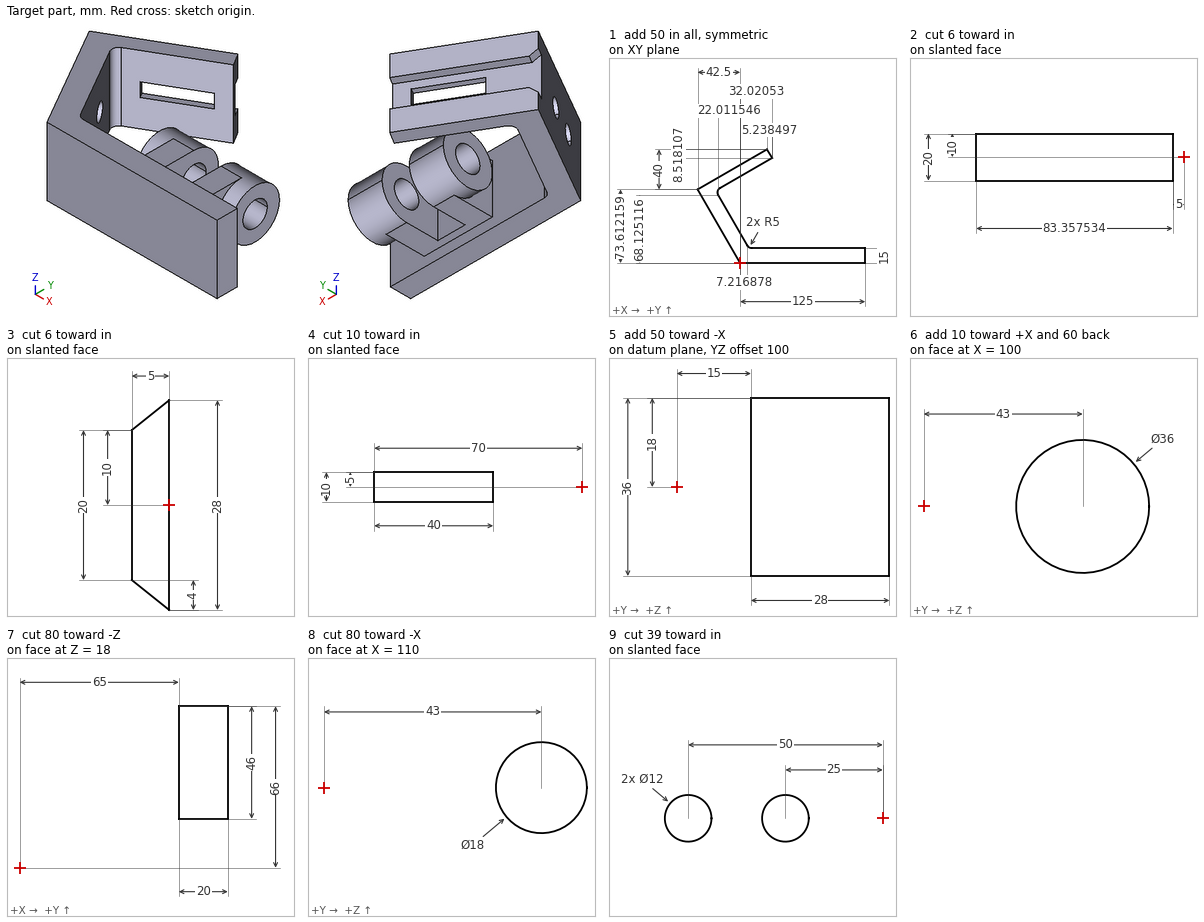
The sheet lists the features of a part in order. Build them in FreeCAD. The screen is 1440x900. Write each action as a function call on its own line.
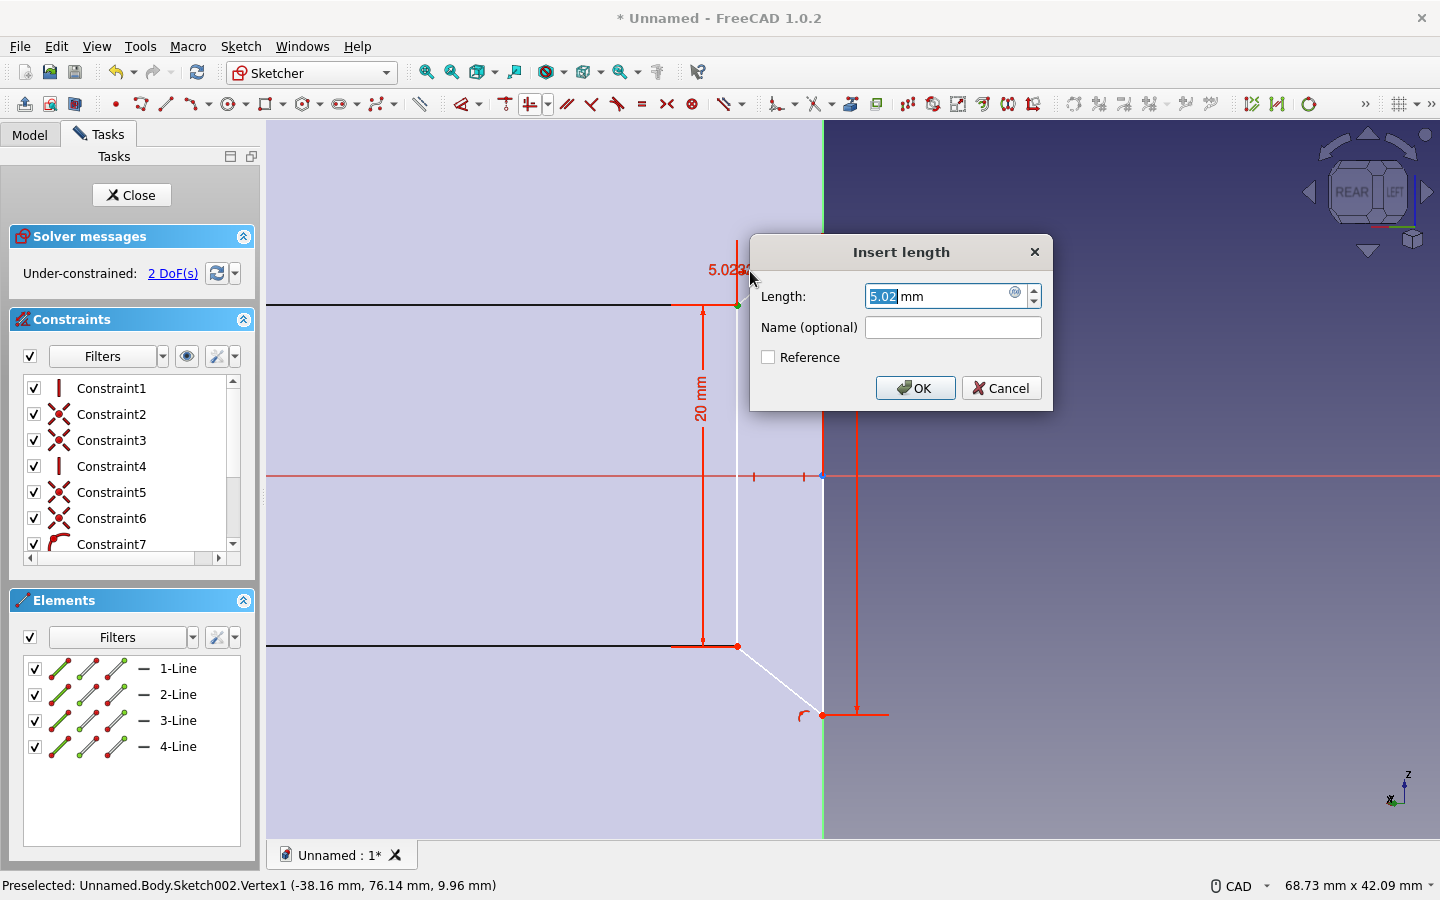
text(5)
key(Return)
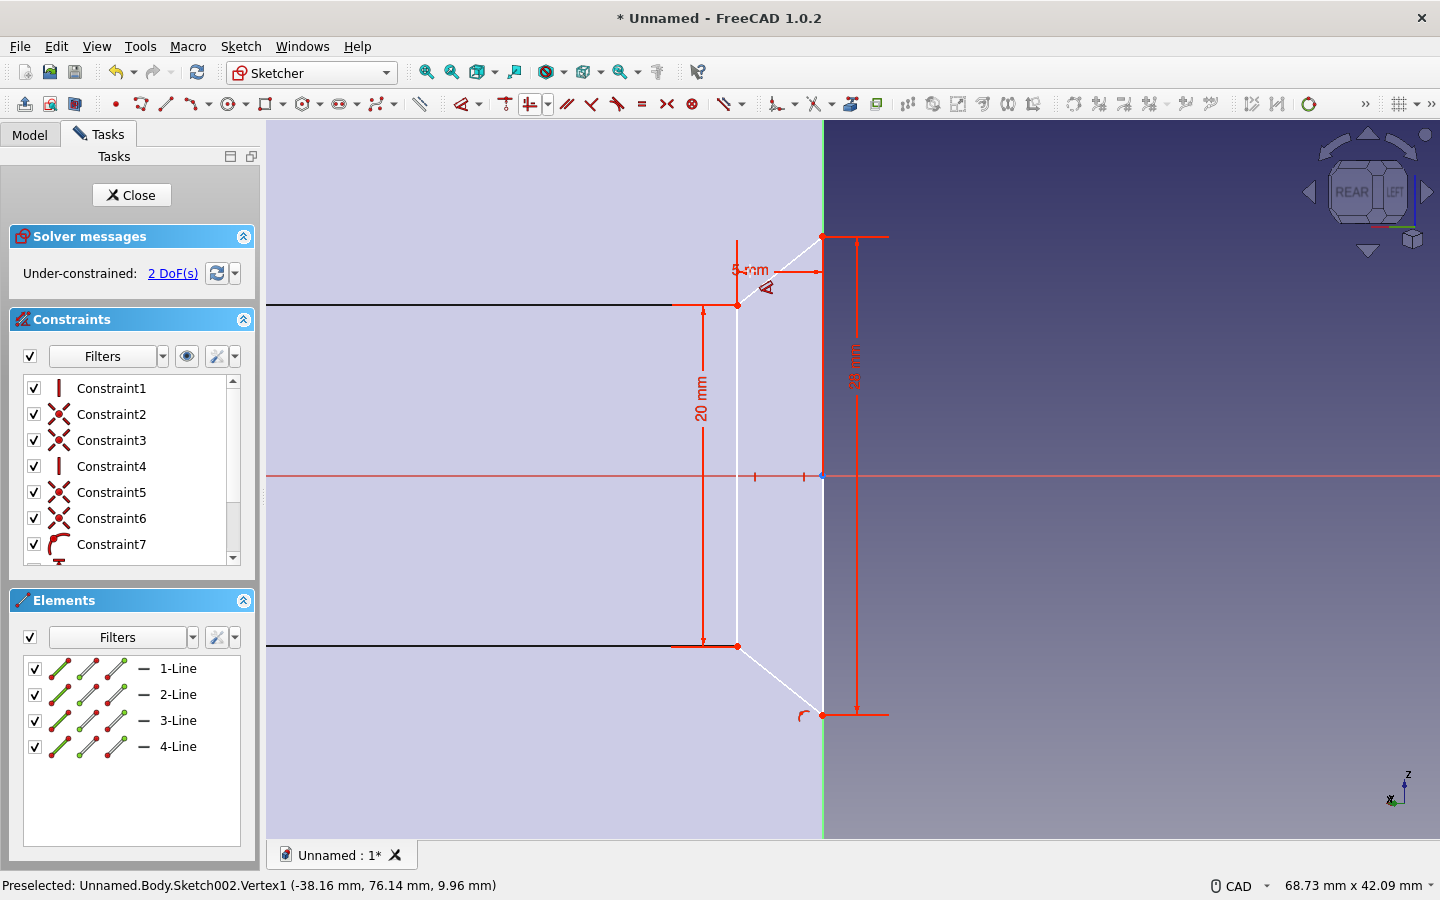
click(763, 667)
click(703, 681)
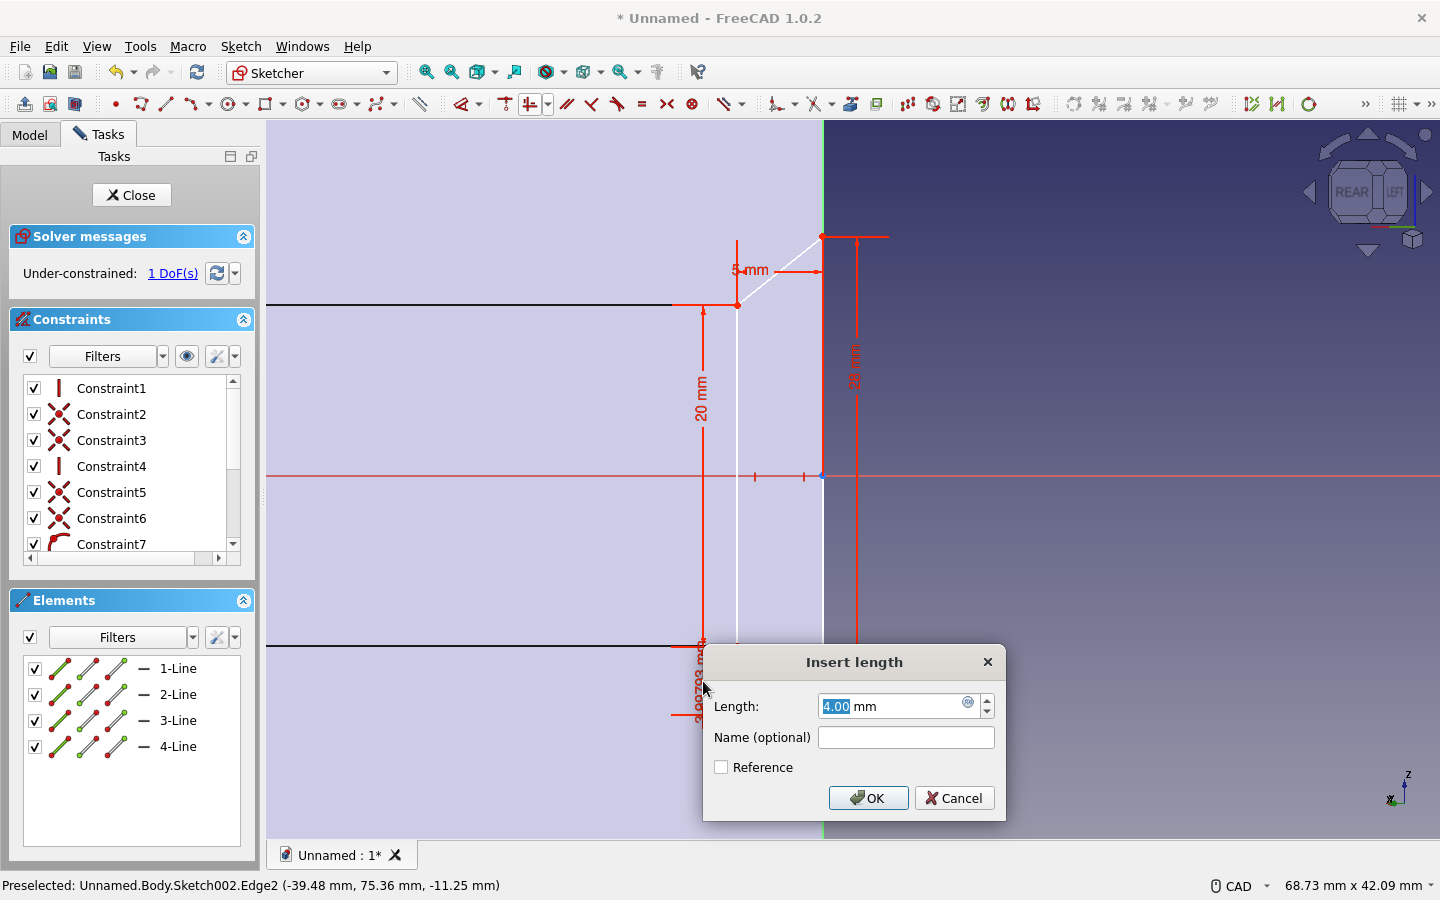
text(4)
key(Return)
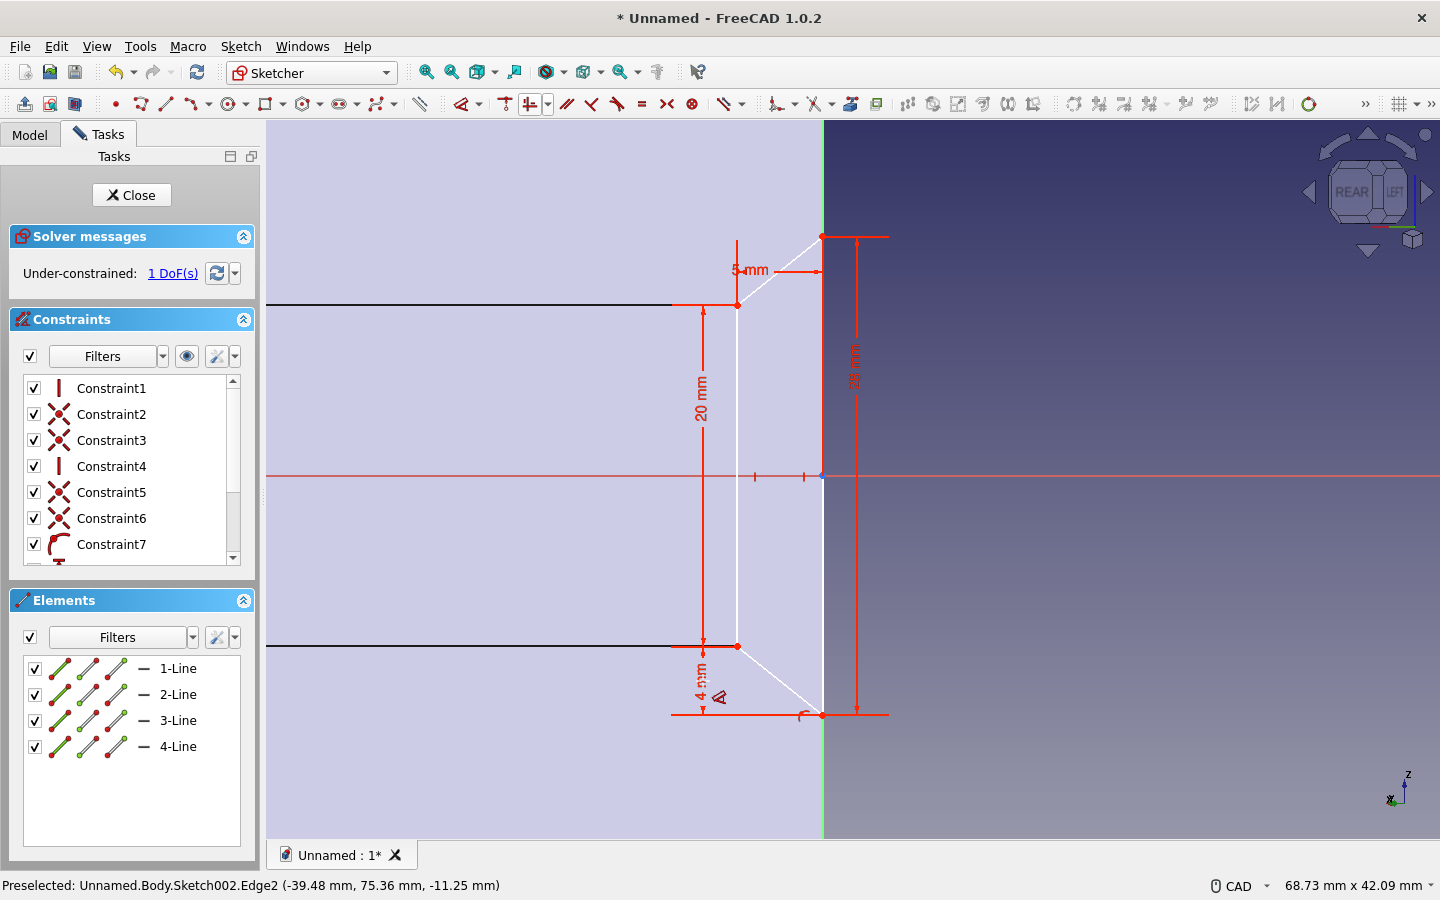
click(737, 305)
click(703, 351)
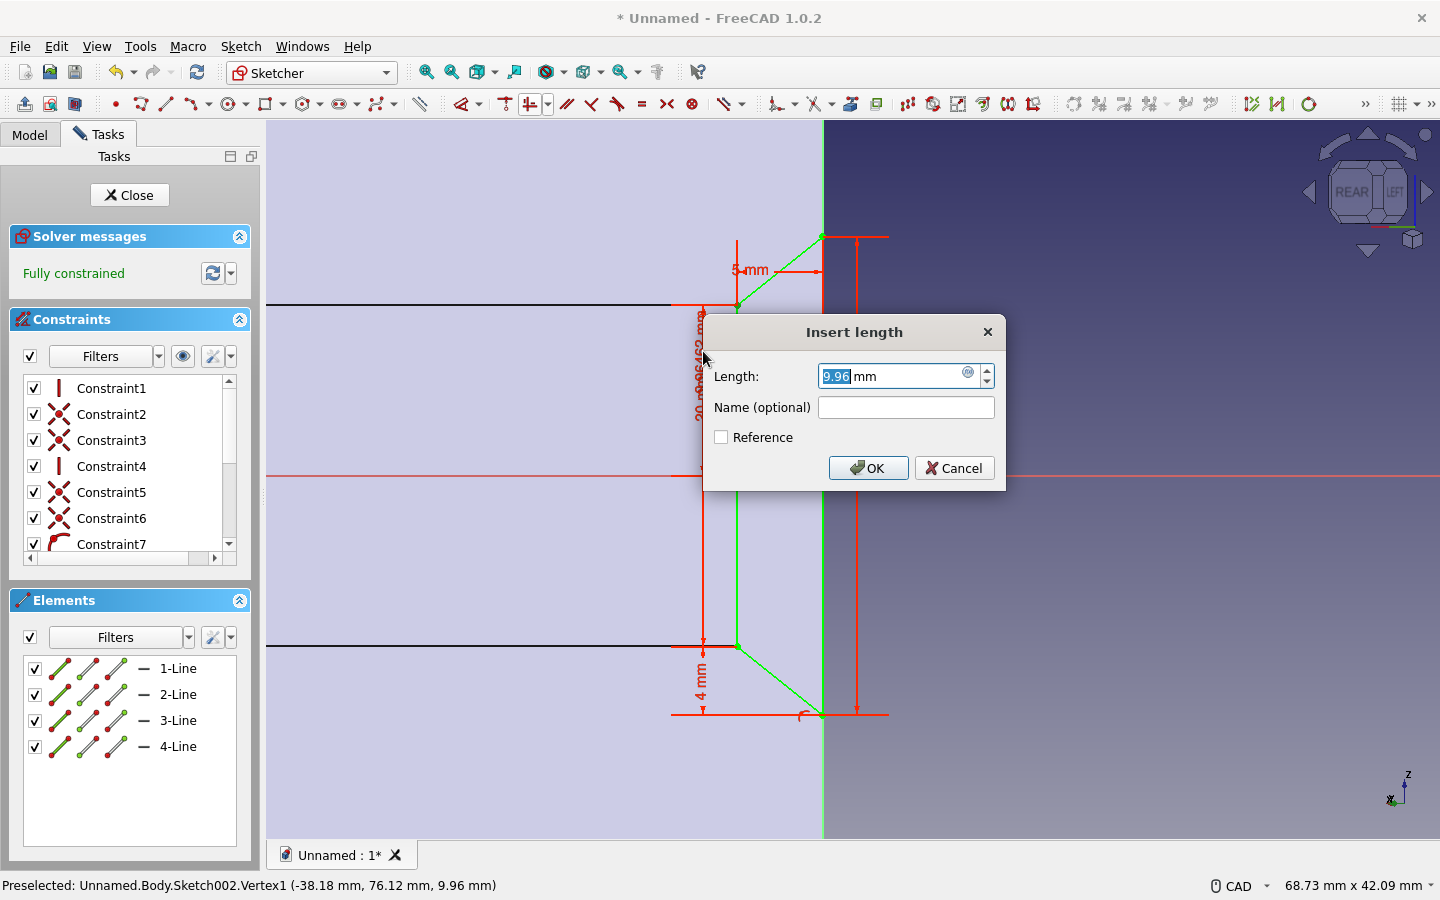
text(10)
key(Return)
key(Escape)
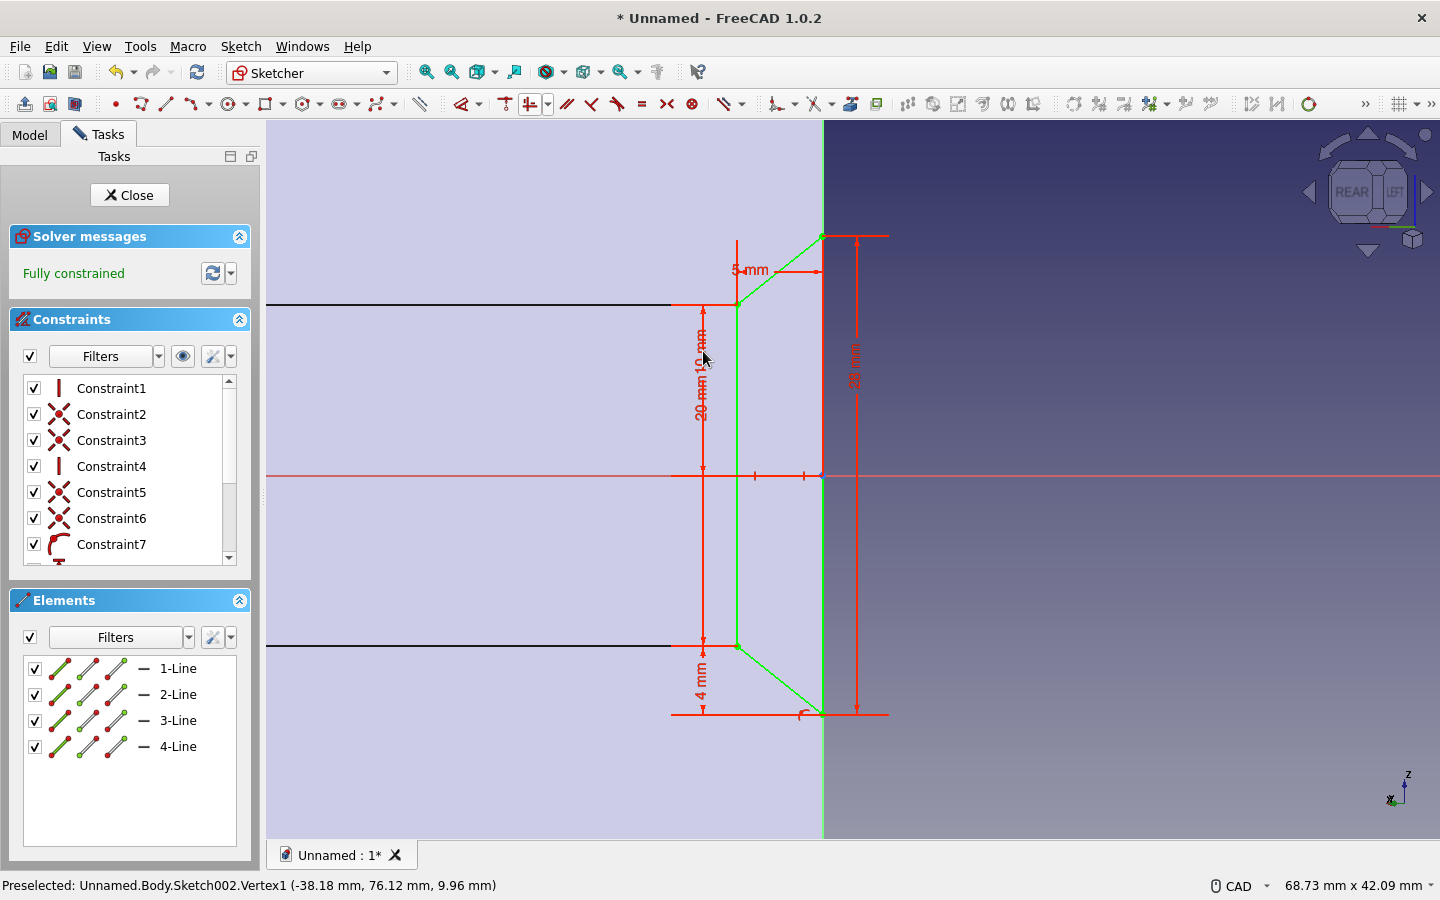
click(130, 195)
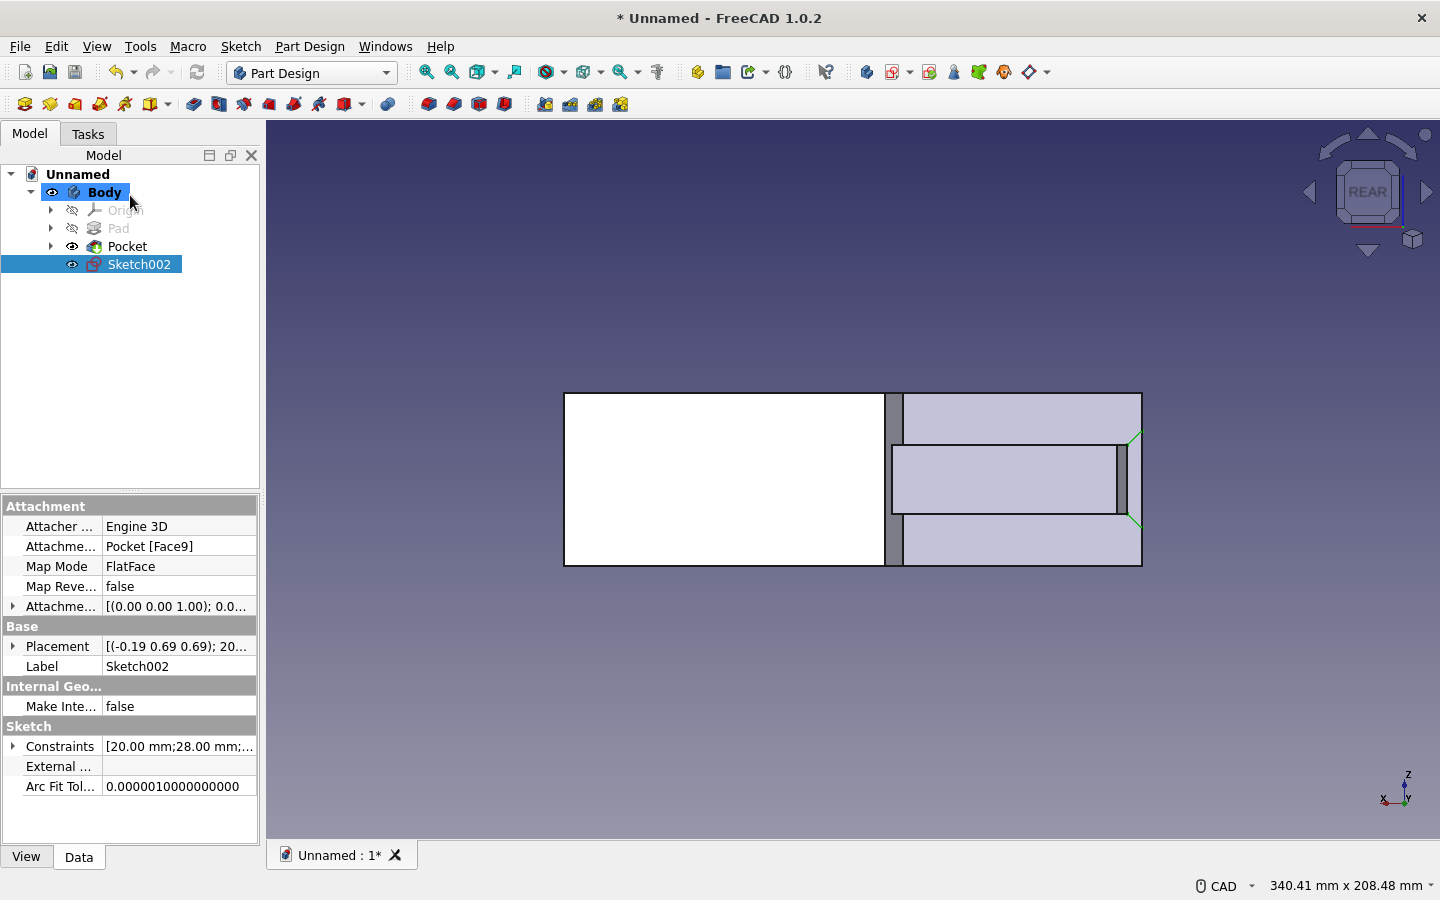
click(194, 104)